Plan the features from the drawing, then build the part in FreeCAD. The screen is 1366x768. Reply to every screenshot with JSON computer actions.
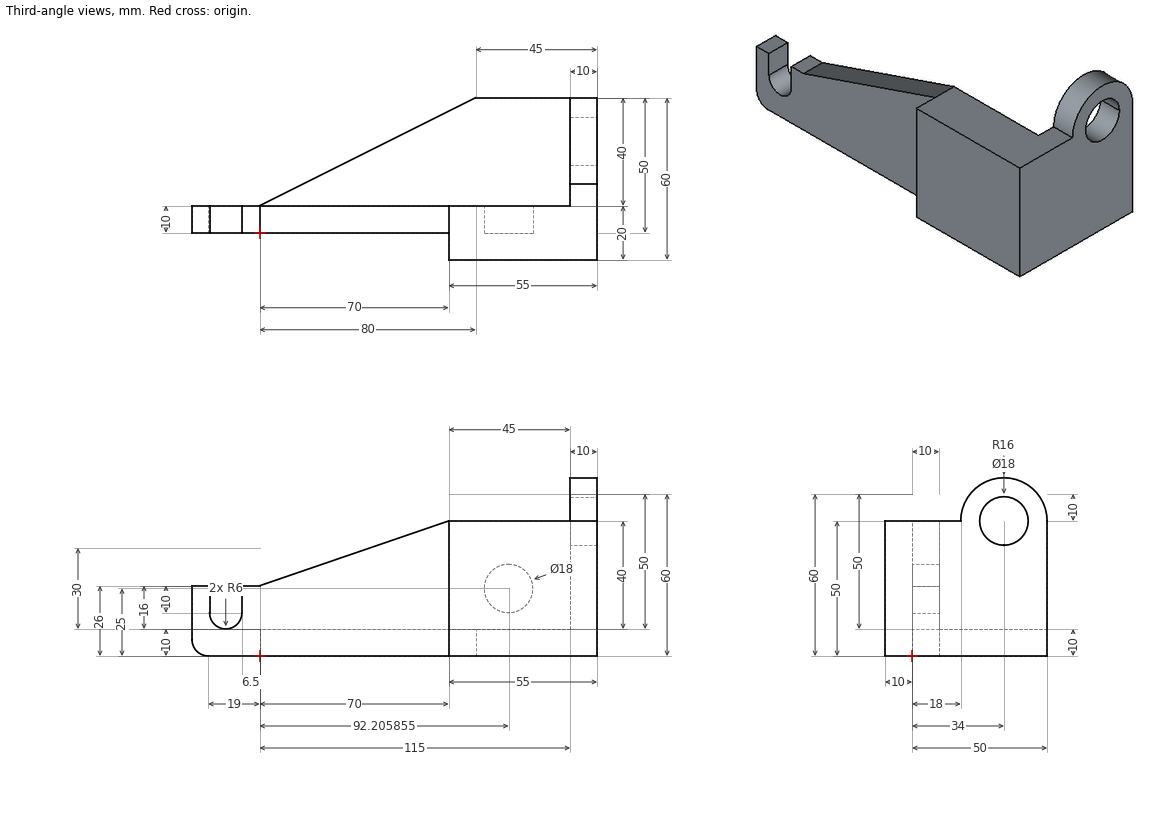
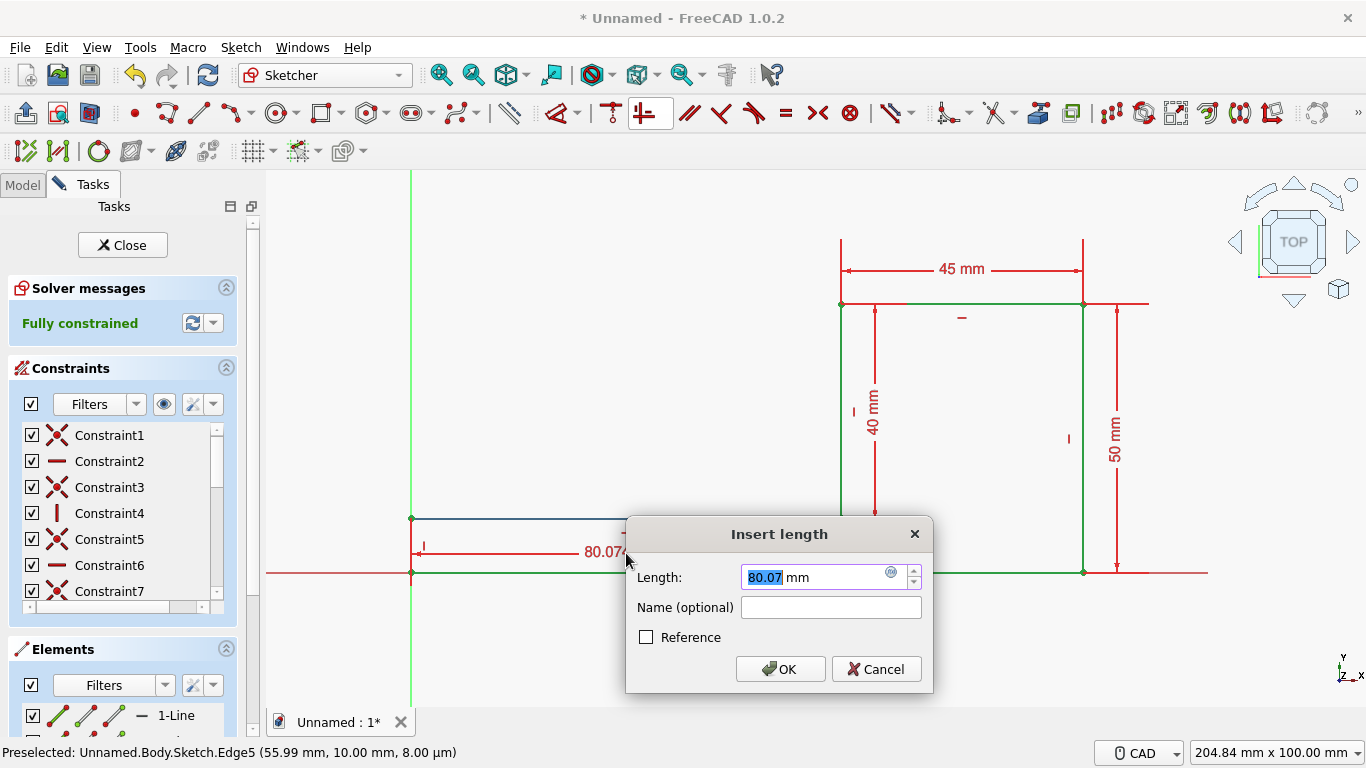
{"action": "type", "text": "80"}
{"action": "key", "text": "Return"}
{"action": "key", "text": "Escape"}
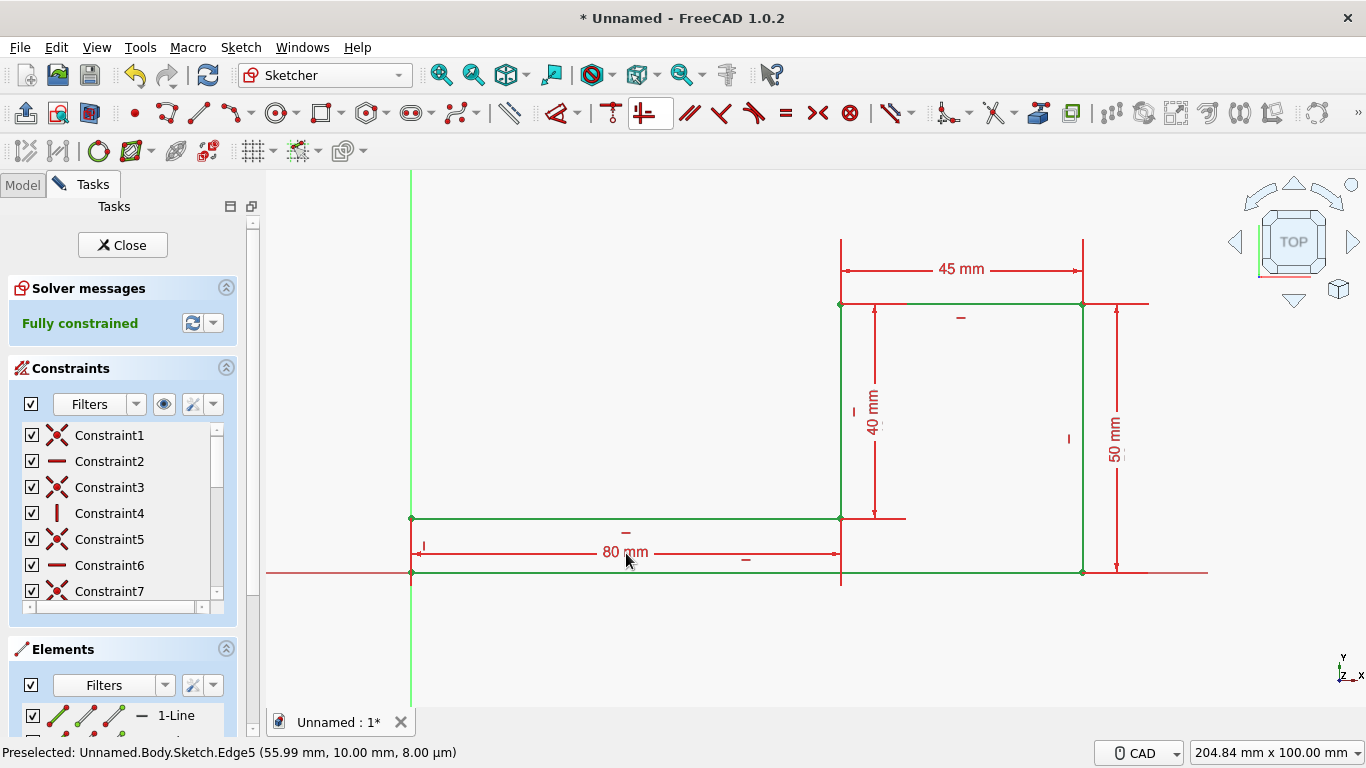
{"action": "left_click", "coordinate": [123, 245]}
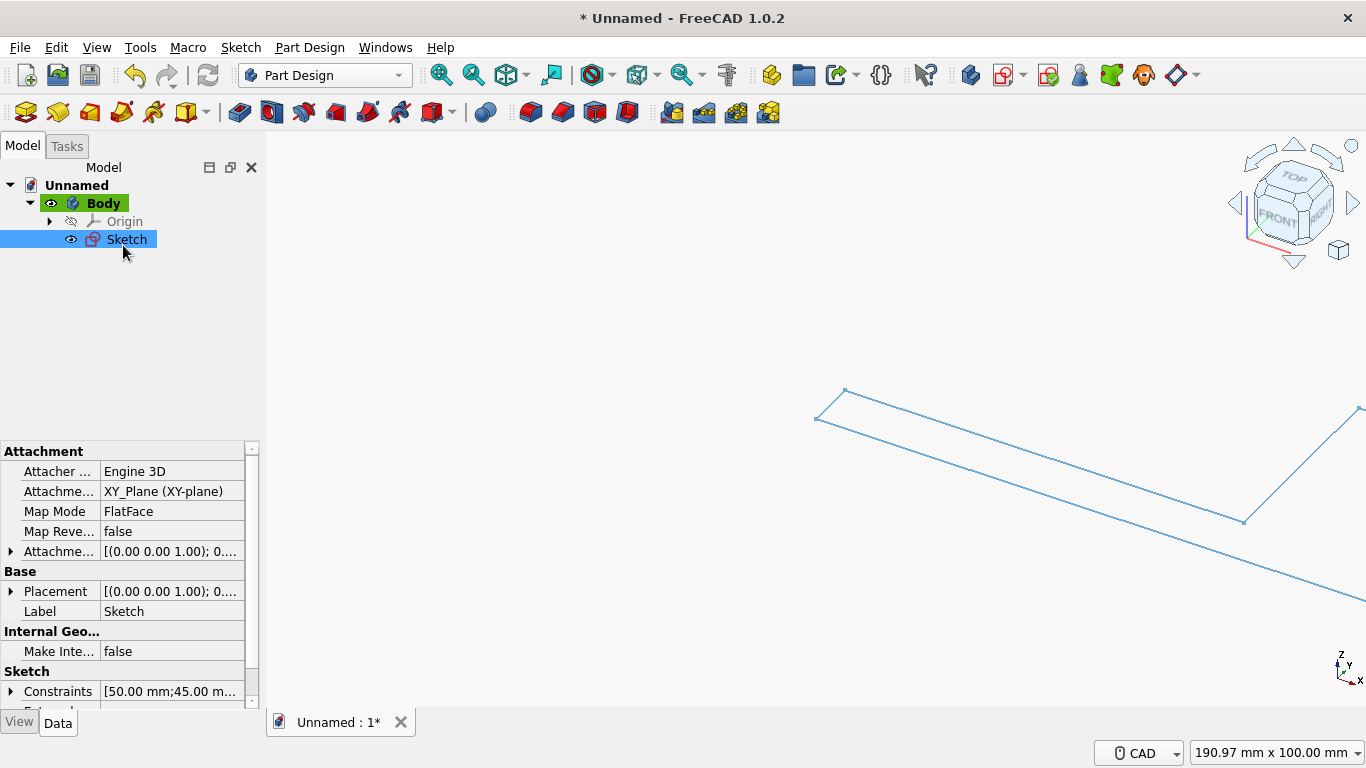
{"action": "left_click", "coordinate": [26, 112]}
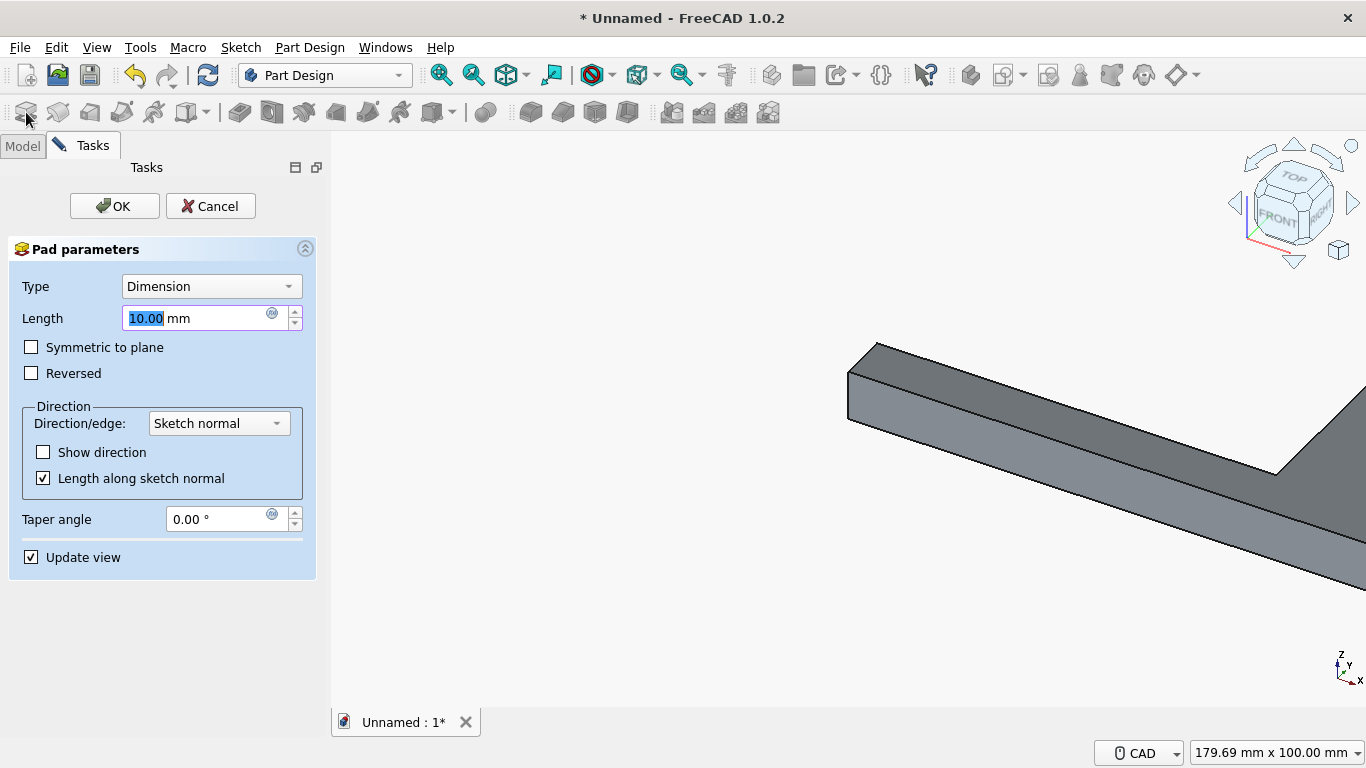
{"action": "type", "text": "10"}
{"action": "key", "text": "Tab"}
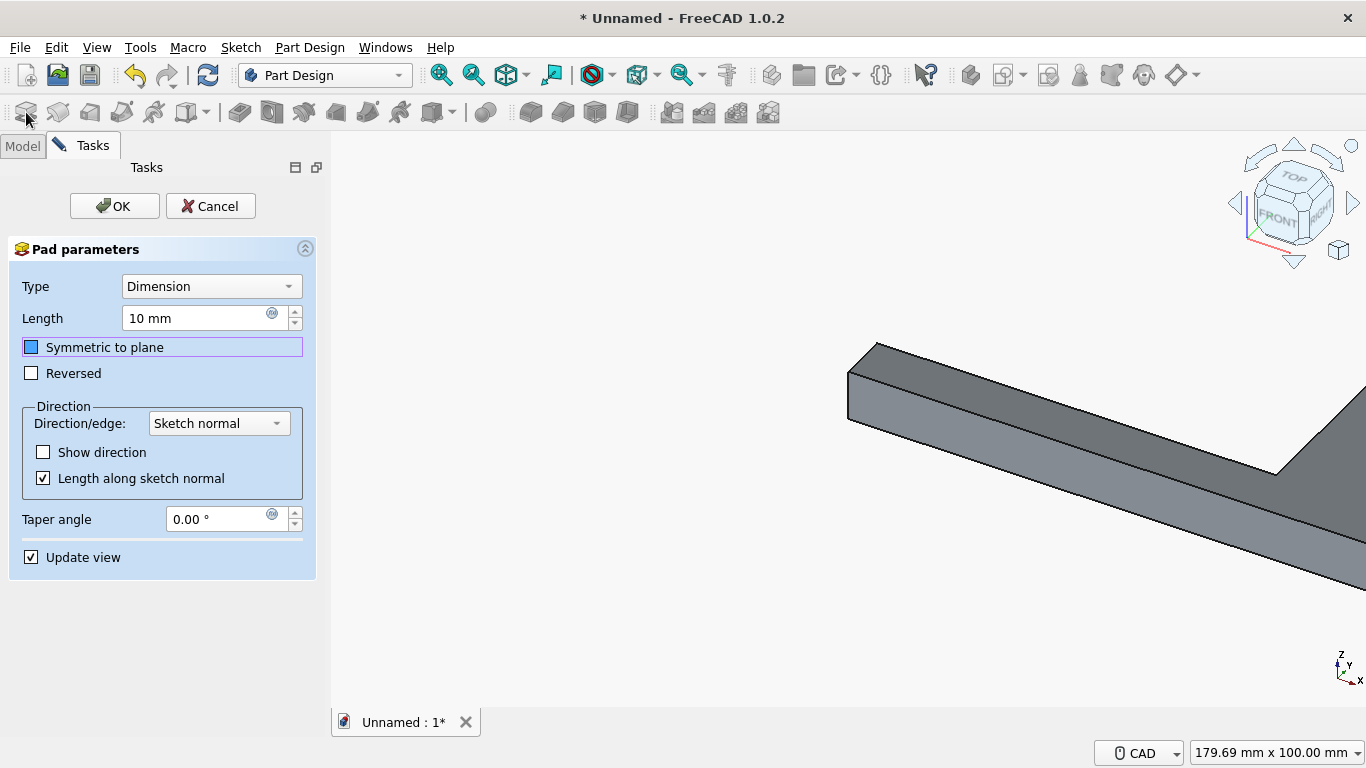
{"action": "left_click", "coordinate": [115, 206]}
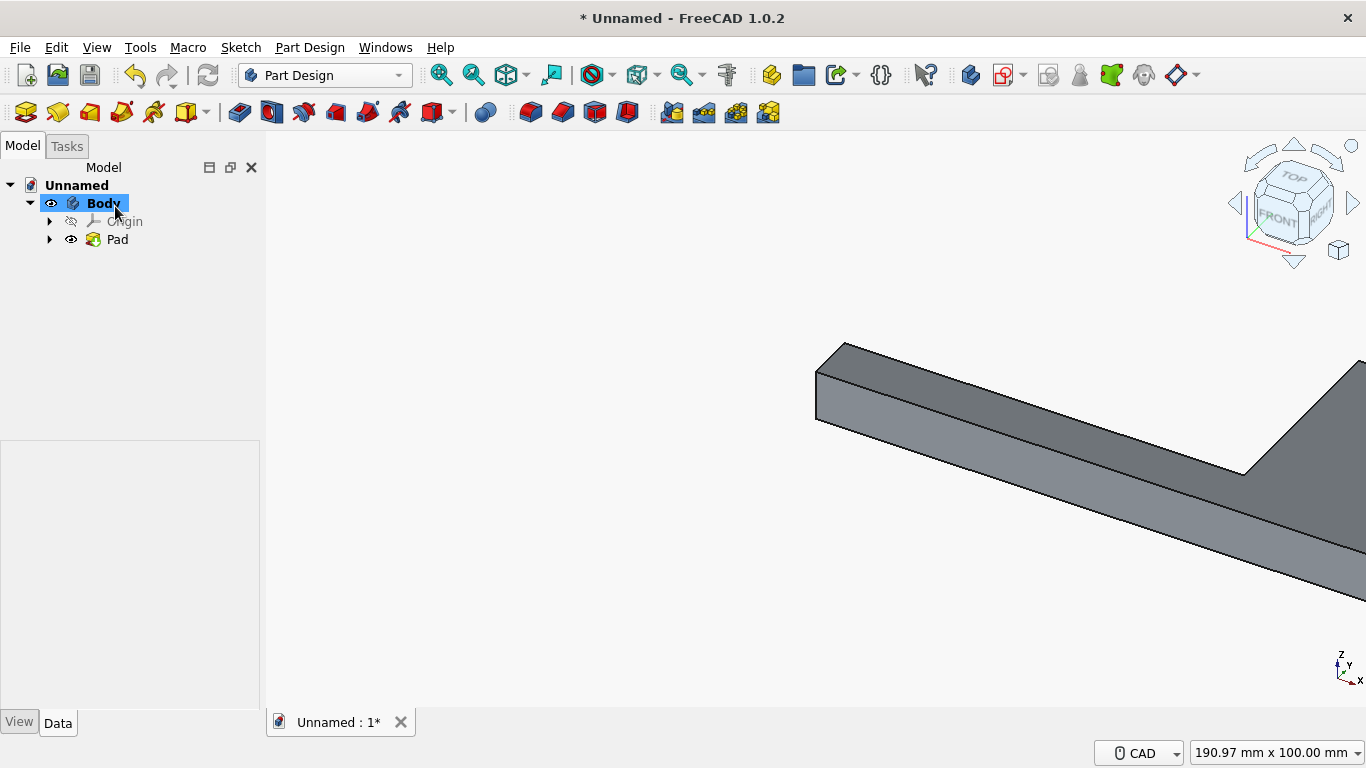
{"action": "left_click", "coordinate": [442, 76]}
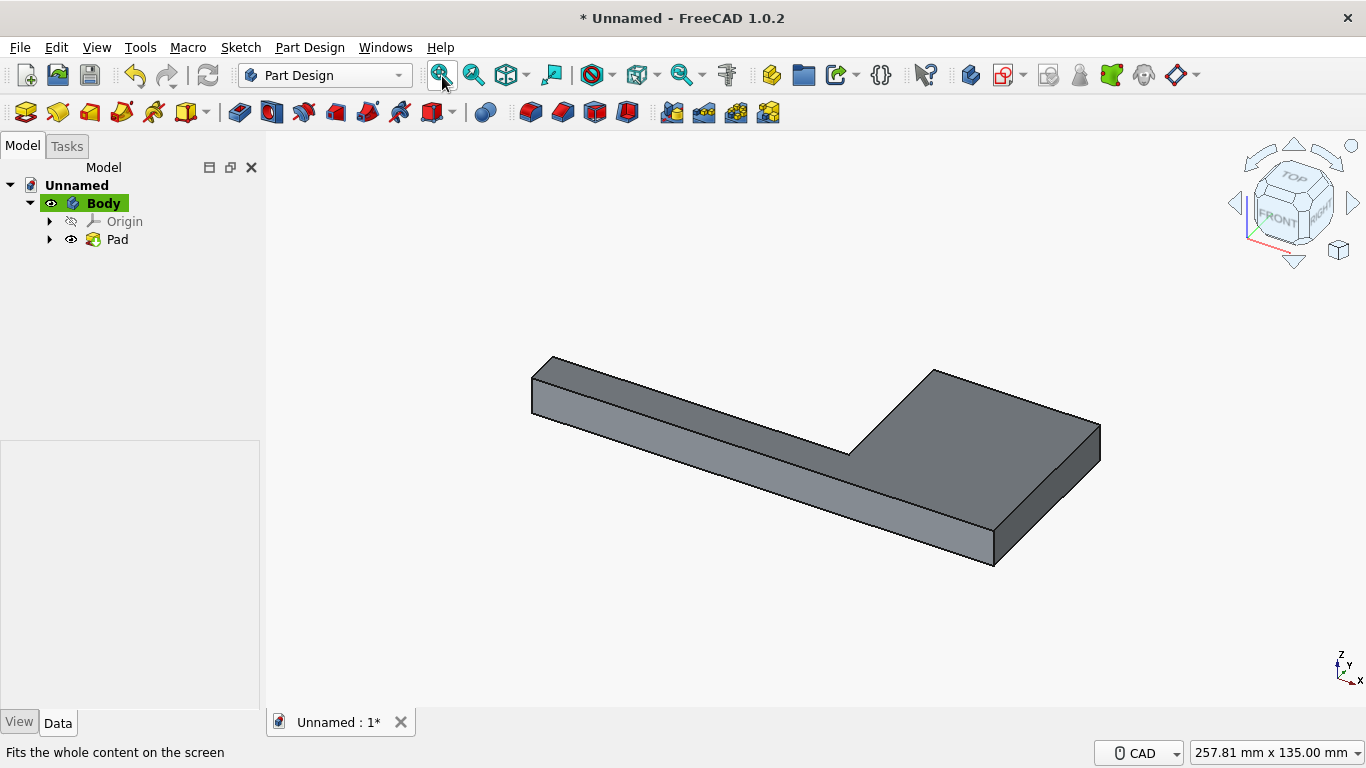
{"action": "left_click", "coordinate": [1077, 464]}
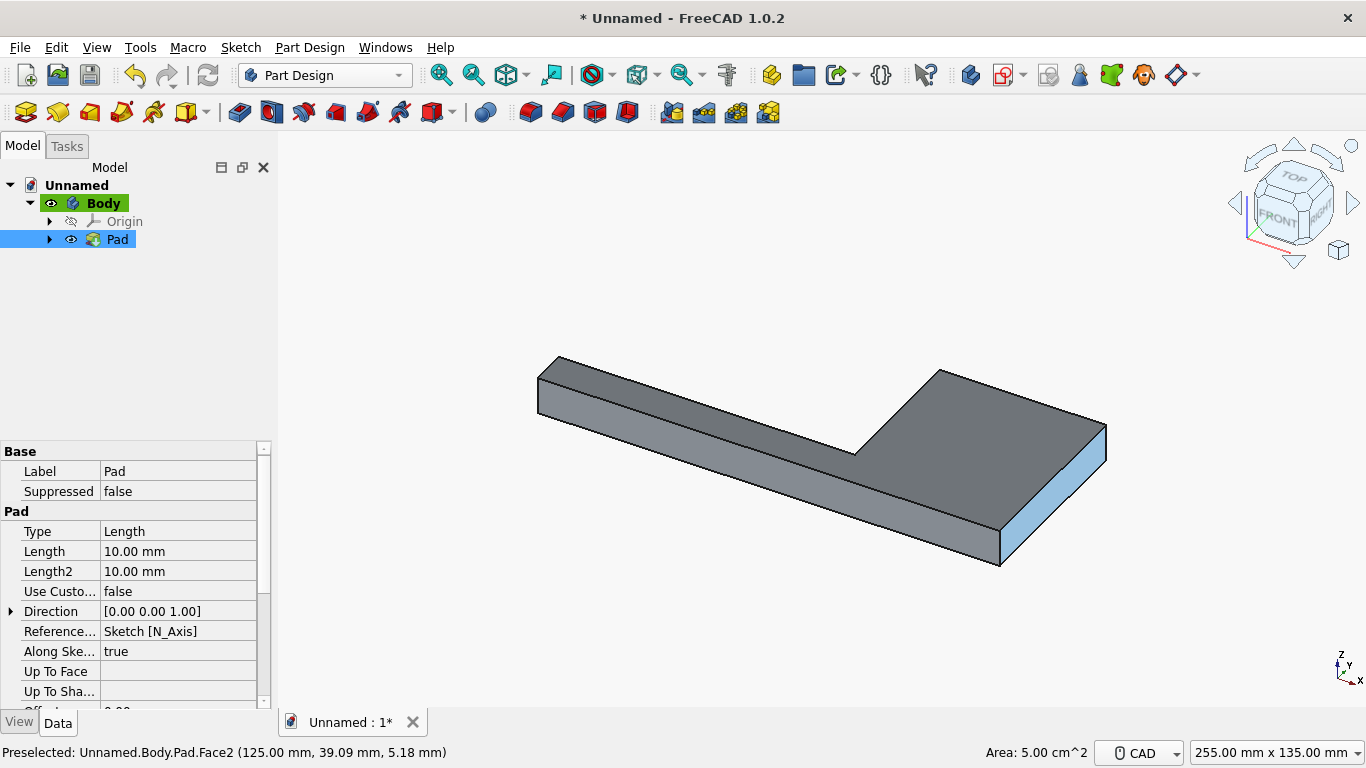
{"action": "left_click", "coordinate": [1004, 76]}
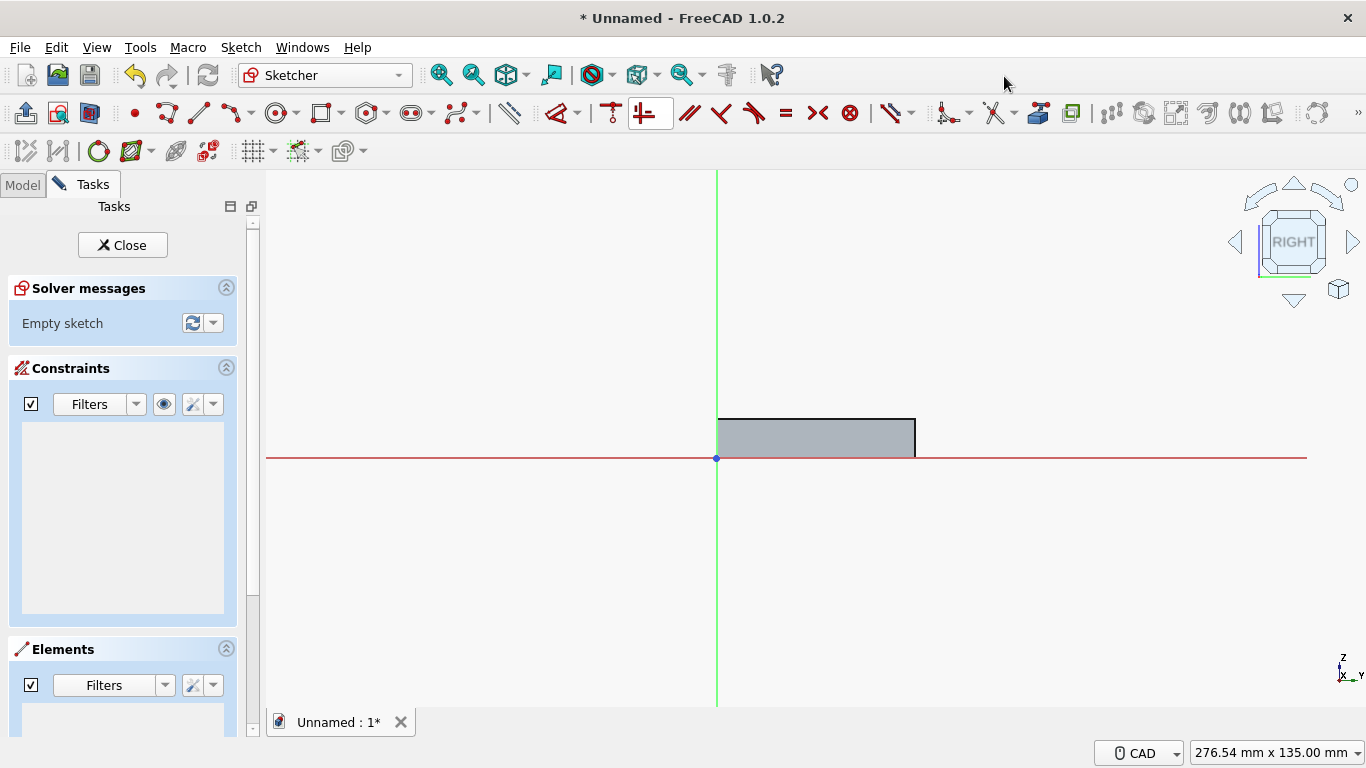
{"action": "scroll", "coordinate": [955, 198], "scroll_direction": "up", "scroll_amount": 2}